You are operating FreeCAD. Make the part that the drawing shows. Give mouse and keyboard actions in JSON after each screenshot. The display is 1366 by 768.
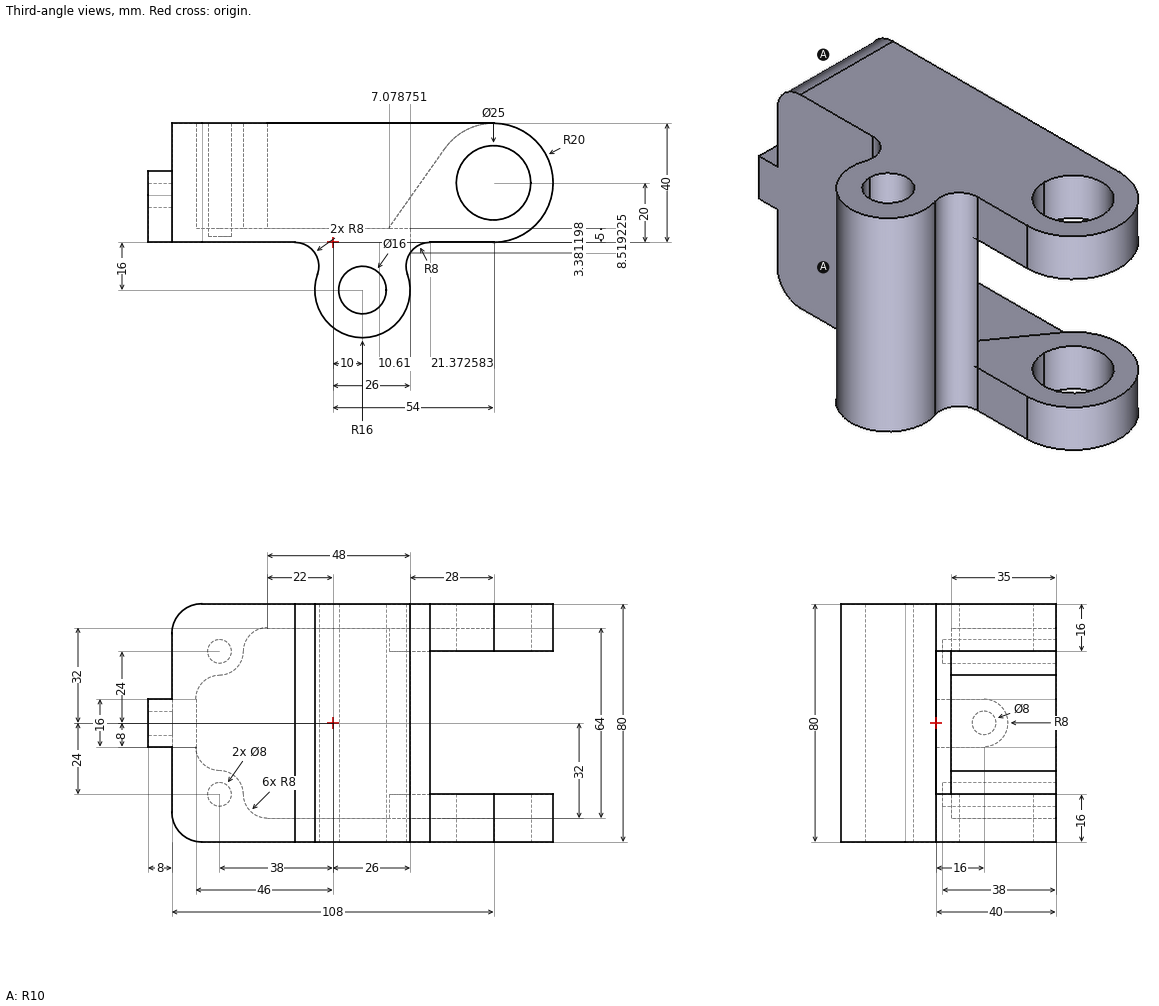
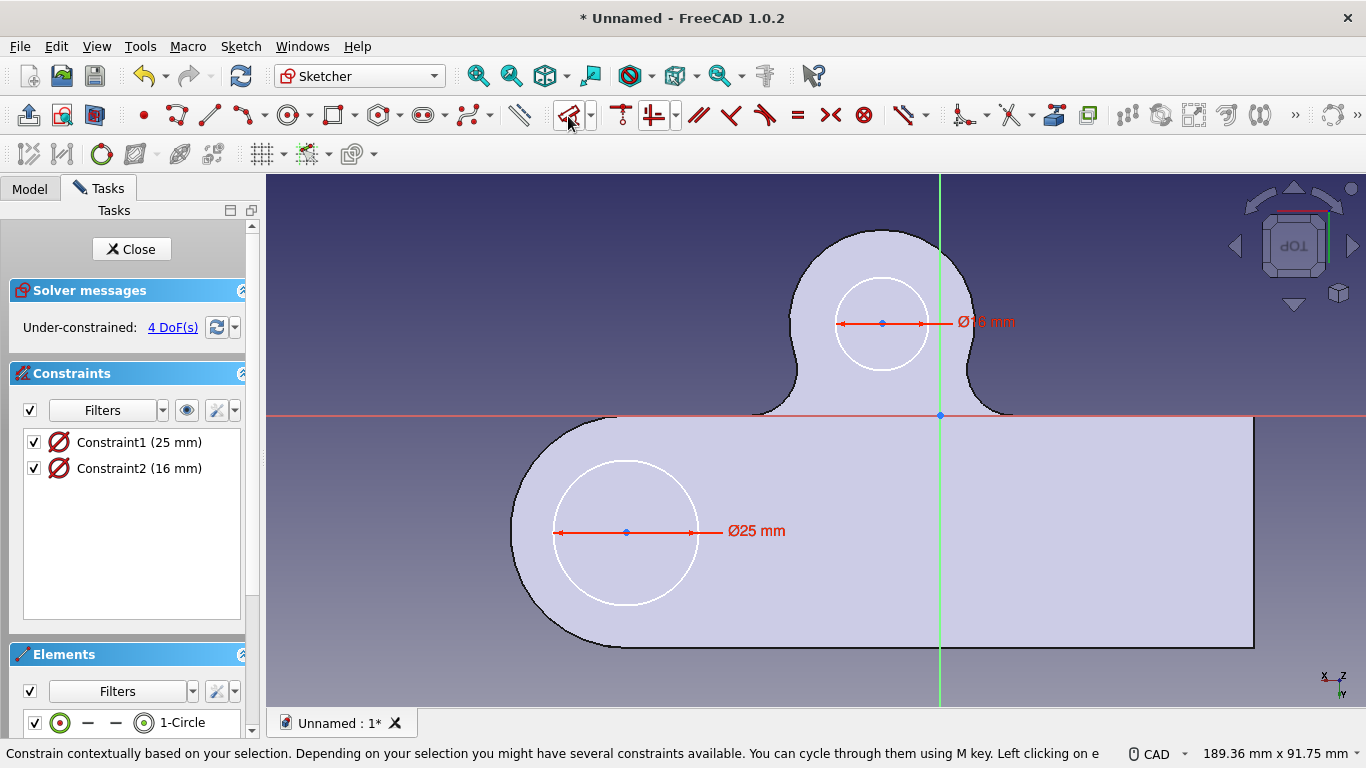
{"action": "left_click", "coordinate": [626, 533]}
{"action": "left_click", "coordinate": [783, 567]}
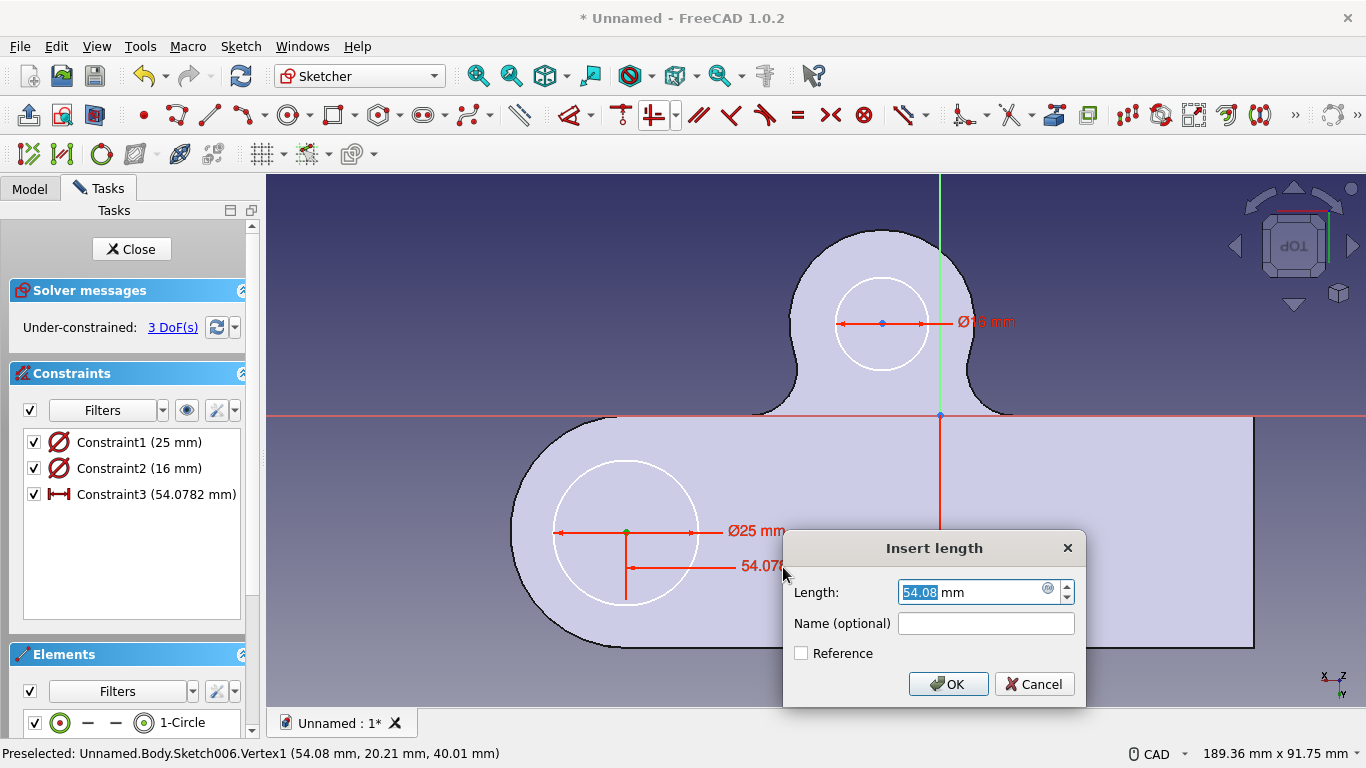
{"action": "type", "text": "54"}
{"action": "key", "text": "Return"}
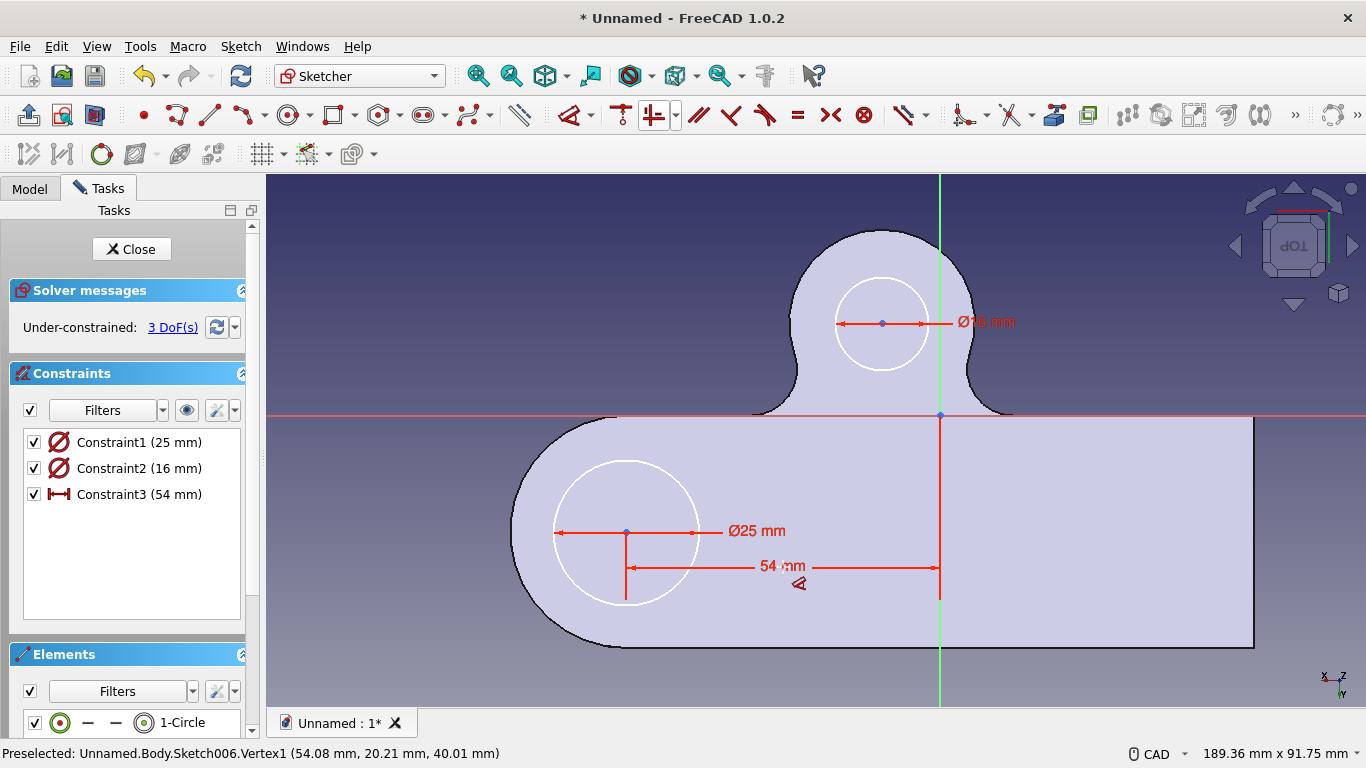
{"action": "left_click", "coordinate": [626, 533]}
{"action": "left_click", "coordinate": [974, 474]}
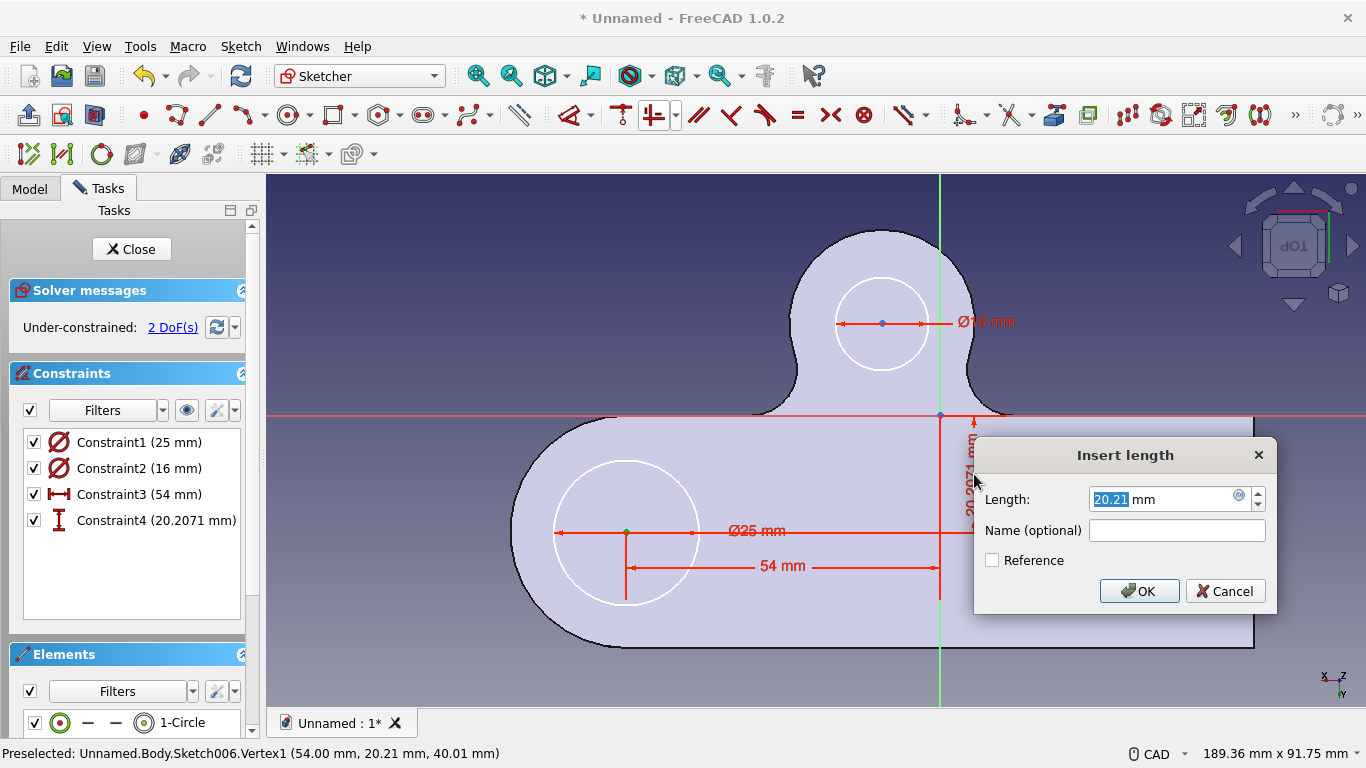
{"action": "type", "text": "20"}
{"action": "key", "text": "Return"}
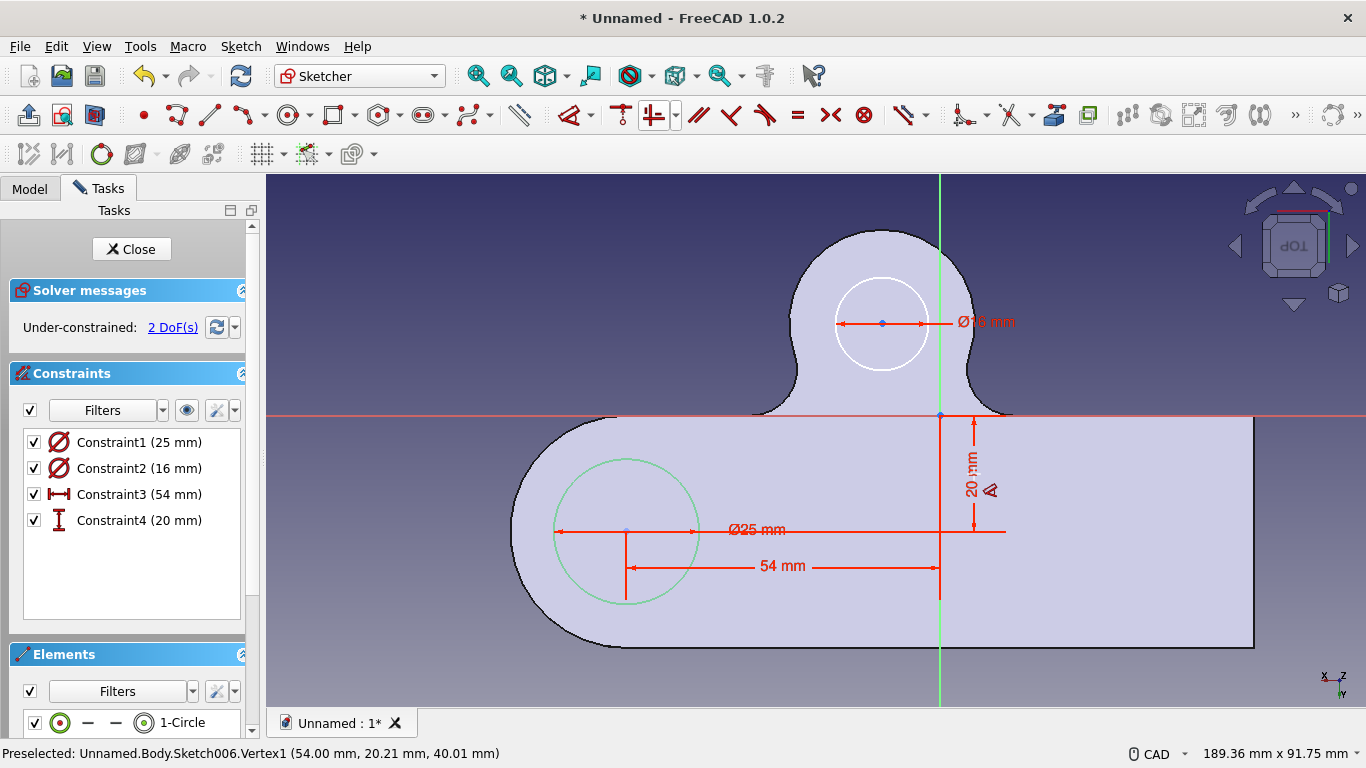
{"action": "left_click", "coordinate": [882, 324]}
{"action": "left_click", "coordinate": [911, 450]}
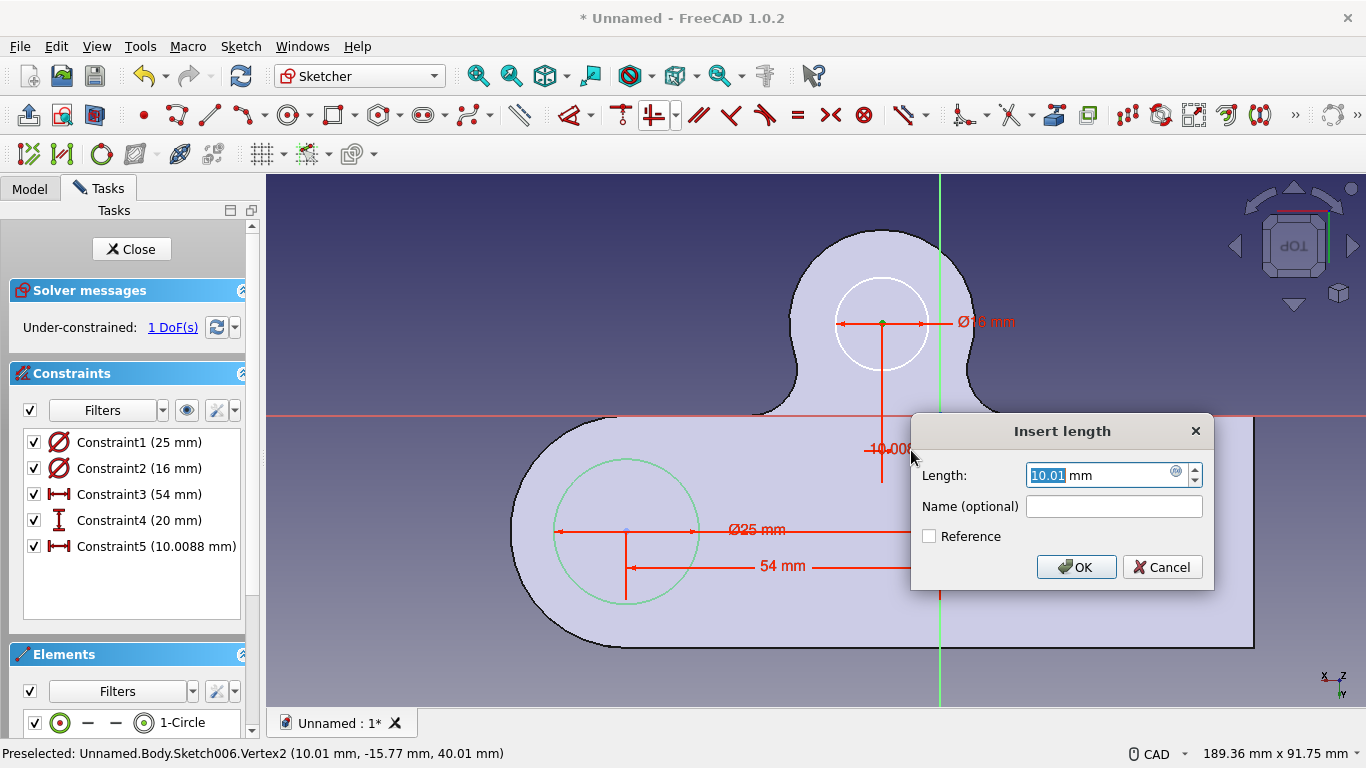
{"action": "type", "text": "10"}
{"action": "key", "text": "Return"}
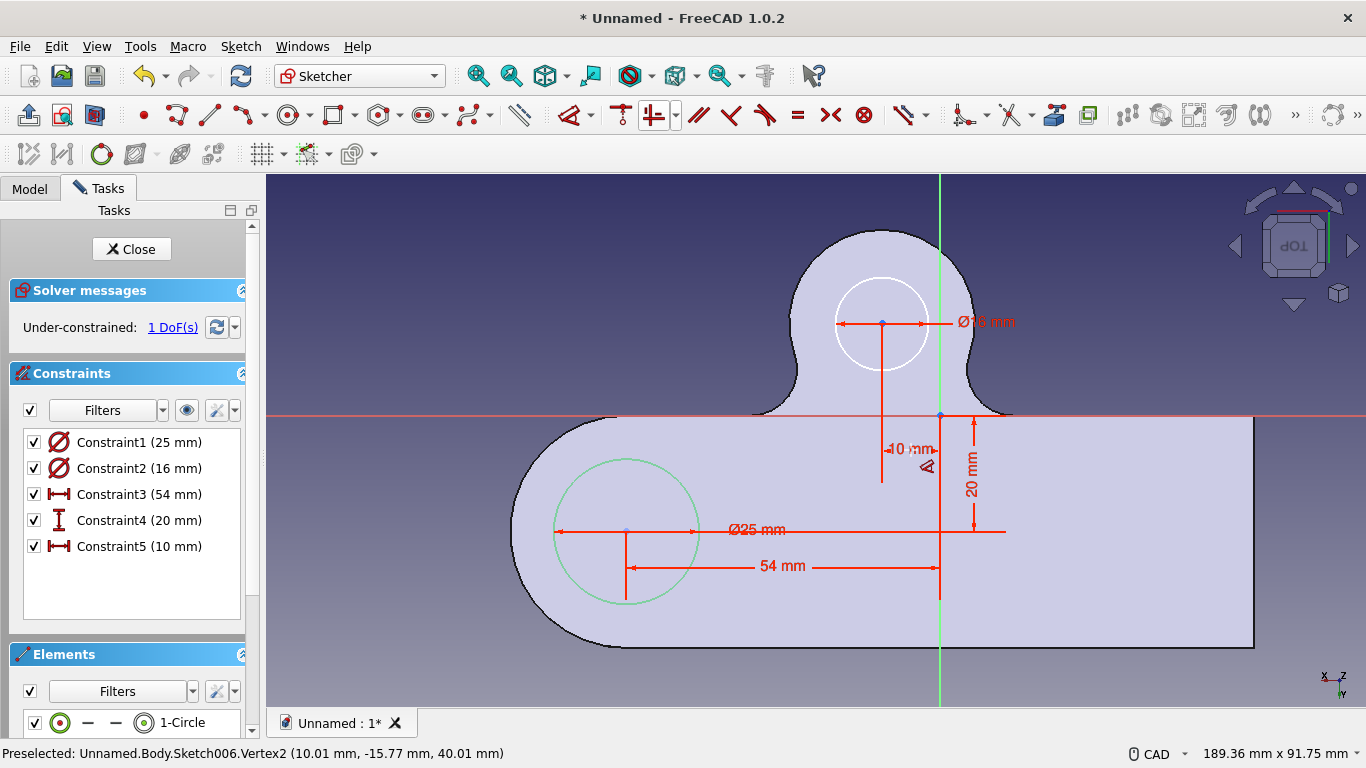
{"action": "left_click", "coordinate": [882, 324]}
{"action": "left_click", "coordinate": [974, 370]}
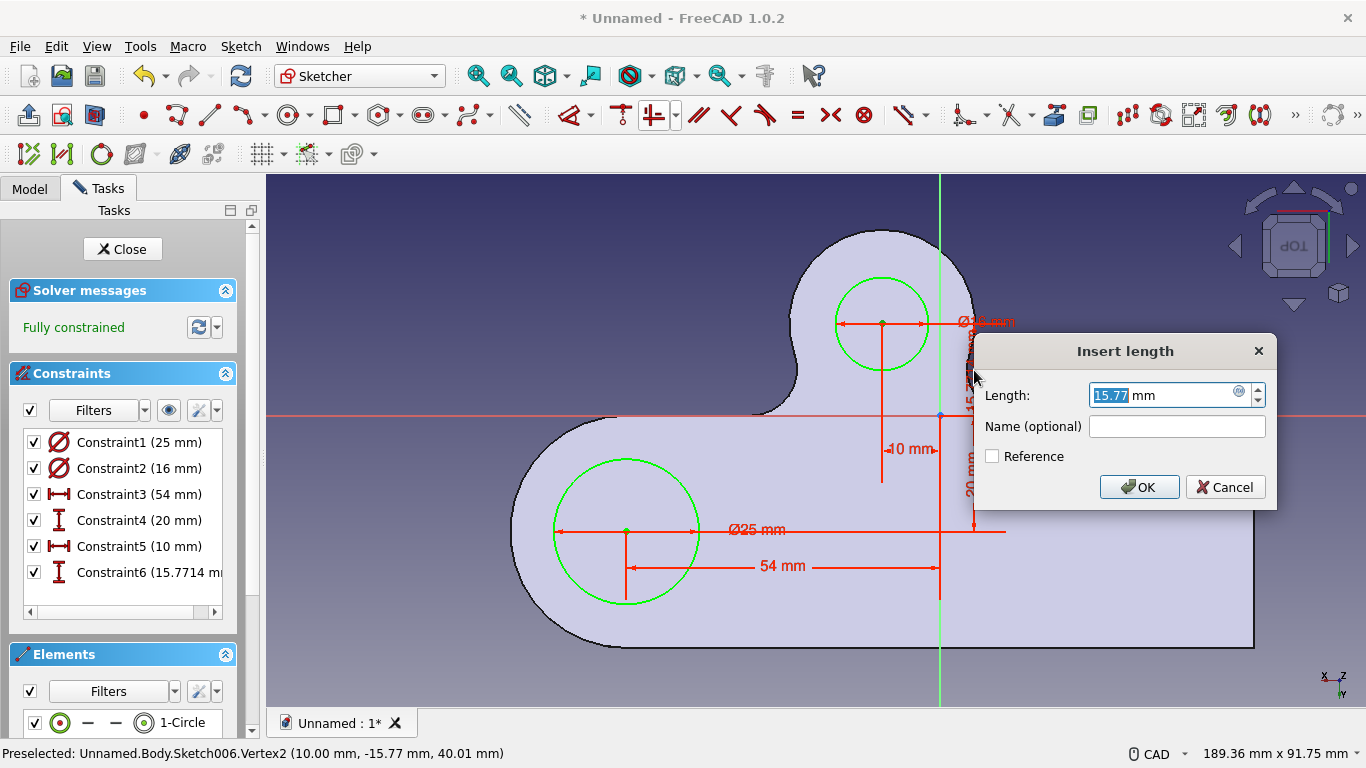
{"action": "type", "text": "16"}
{"action": "key", "text": "Return"}
{"action": "key", "text": "Escape"}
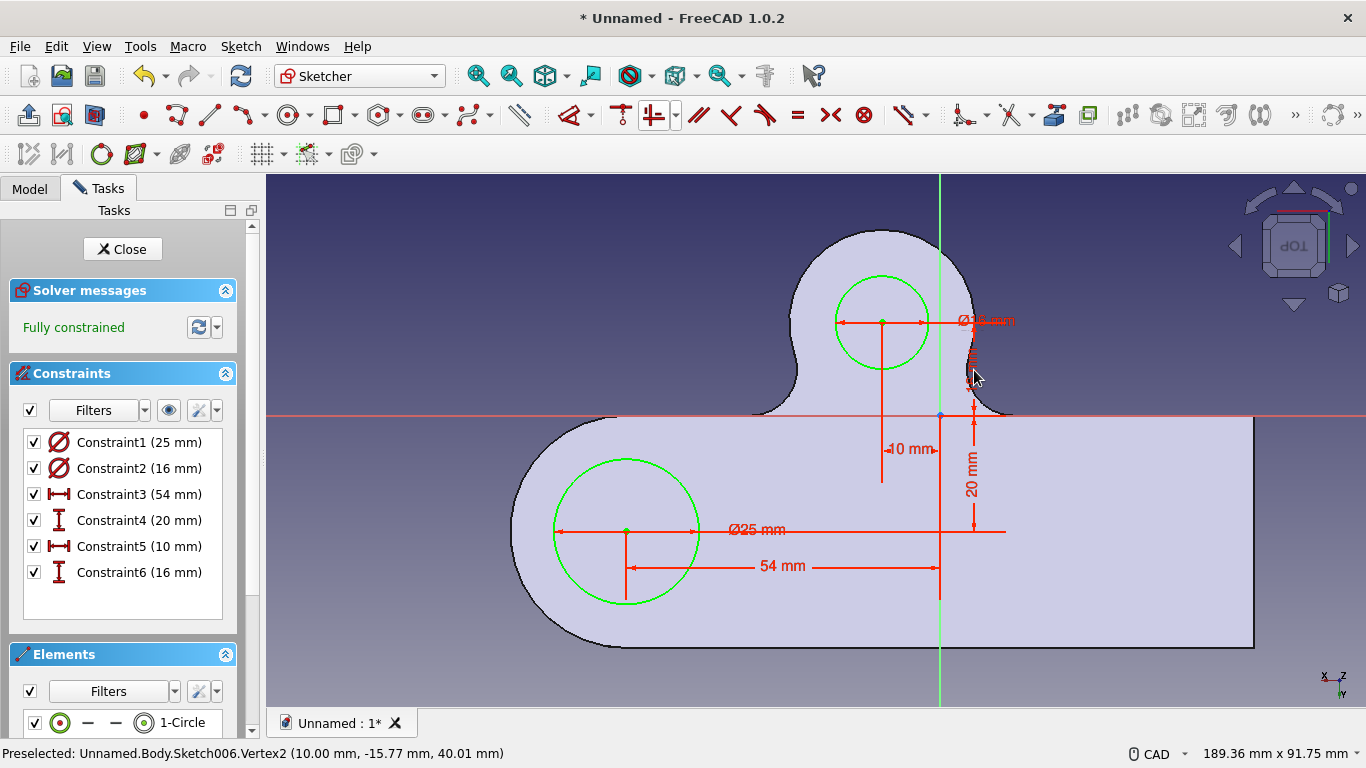
{"action": "left_click", "coordinate": [123, 249]}